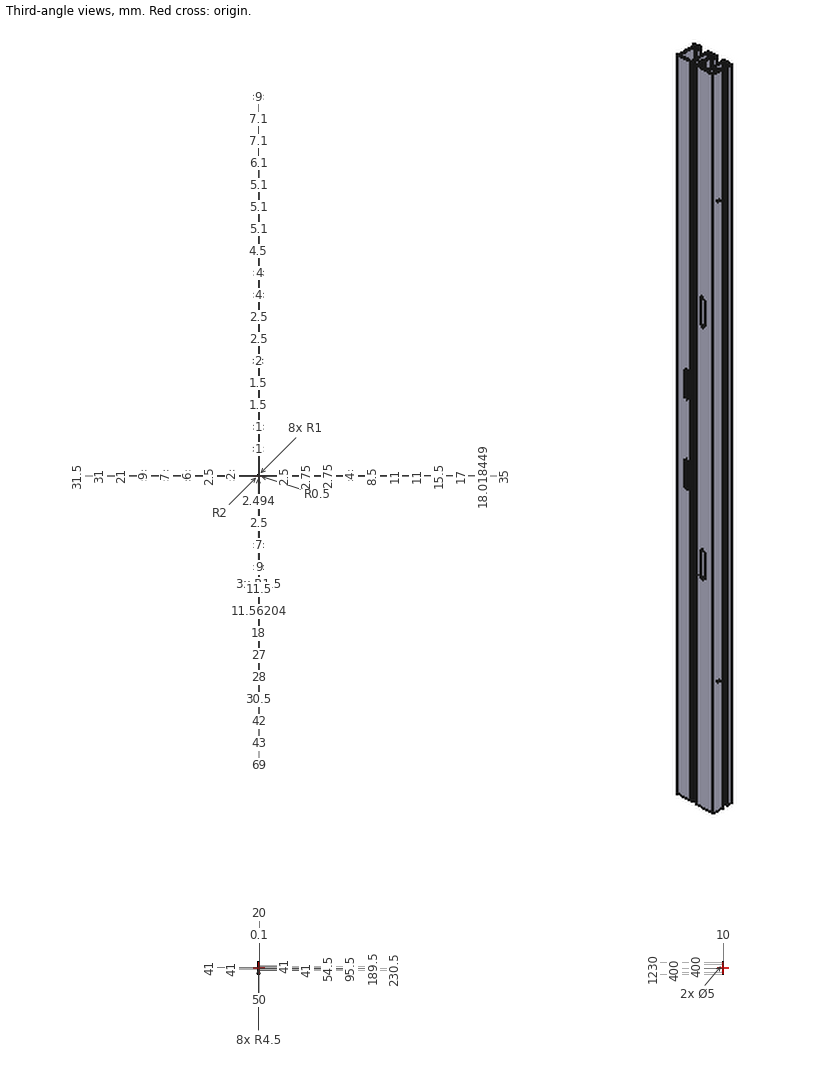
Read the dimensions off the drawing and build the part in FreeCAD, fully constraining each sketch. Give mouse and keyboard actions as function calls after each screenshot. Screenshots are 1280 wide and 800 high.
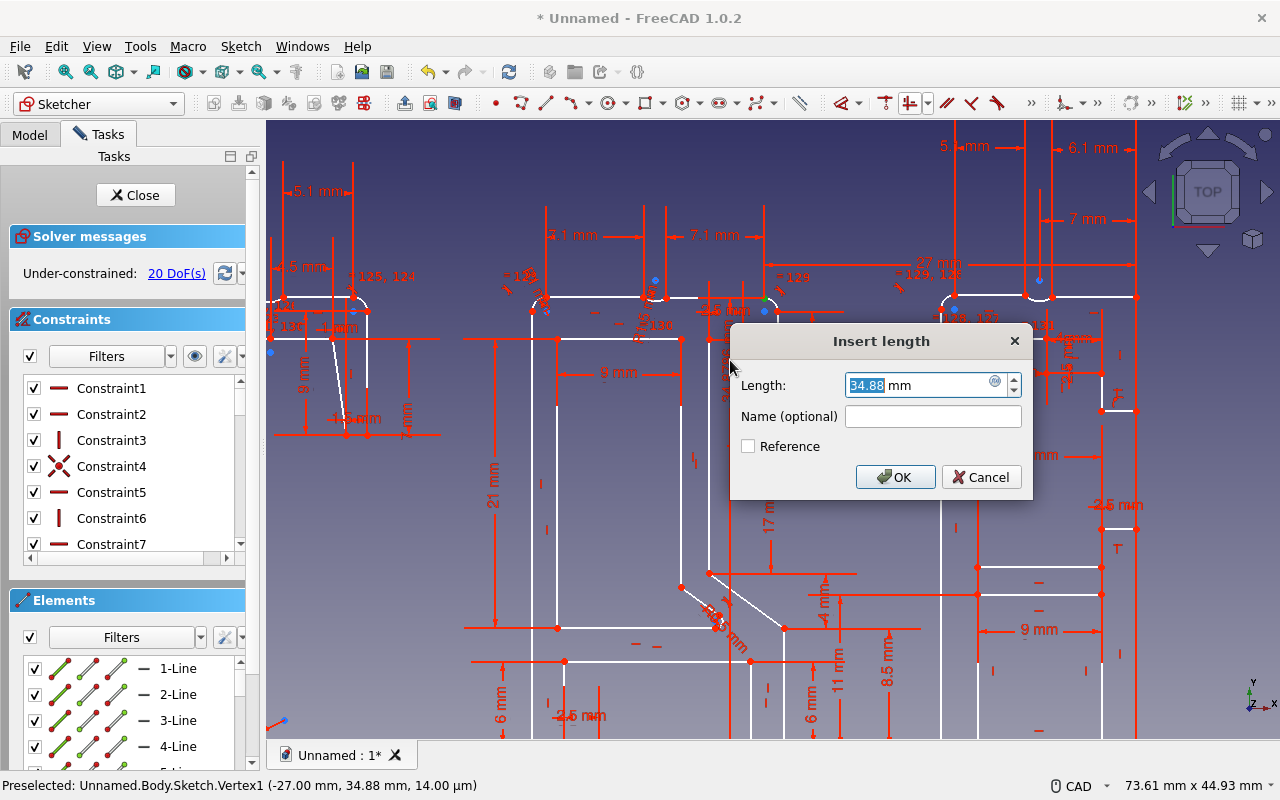
text(35)
key(Return)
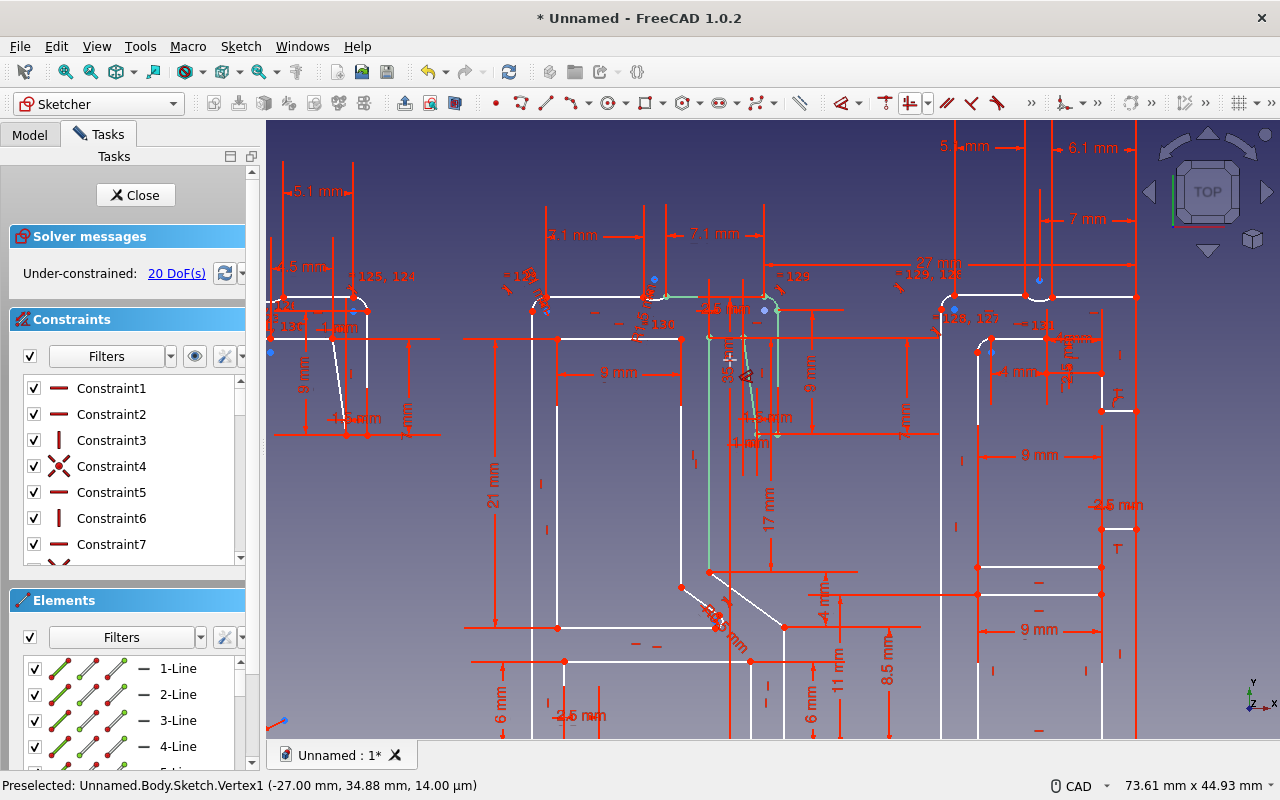
click(644, 297)
click(610, 504)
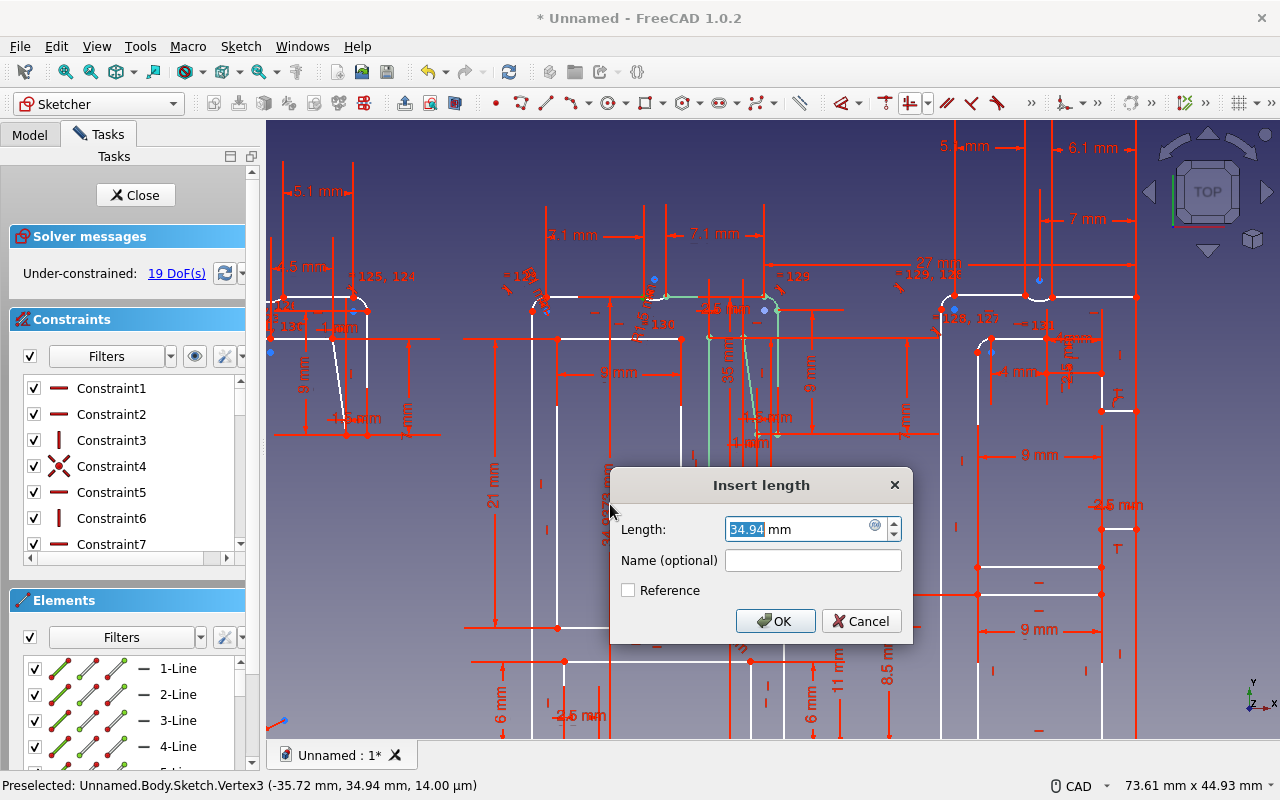
text(35)
key(Return)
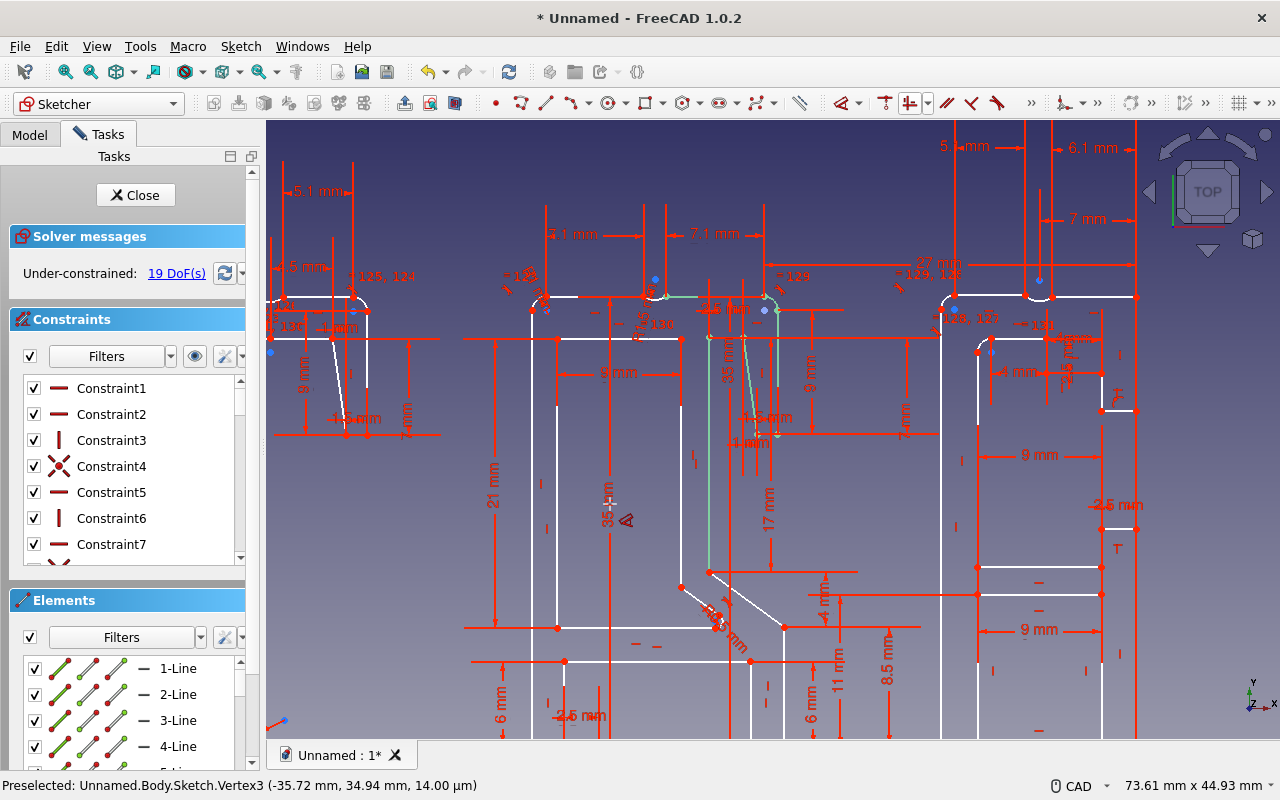
click(546, 297)
click(831, 263)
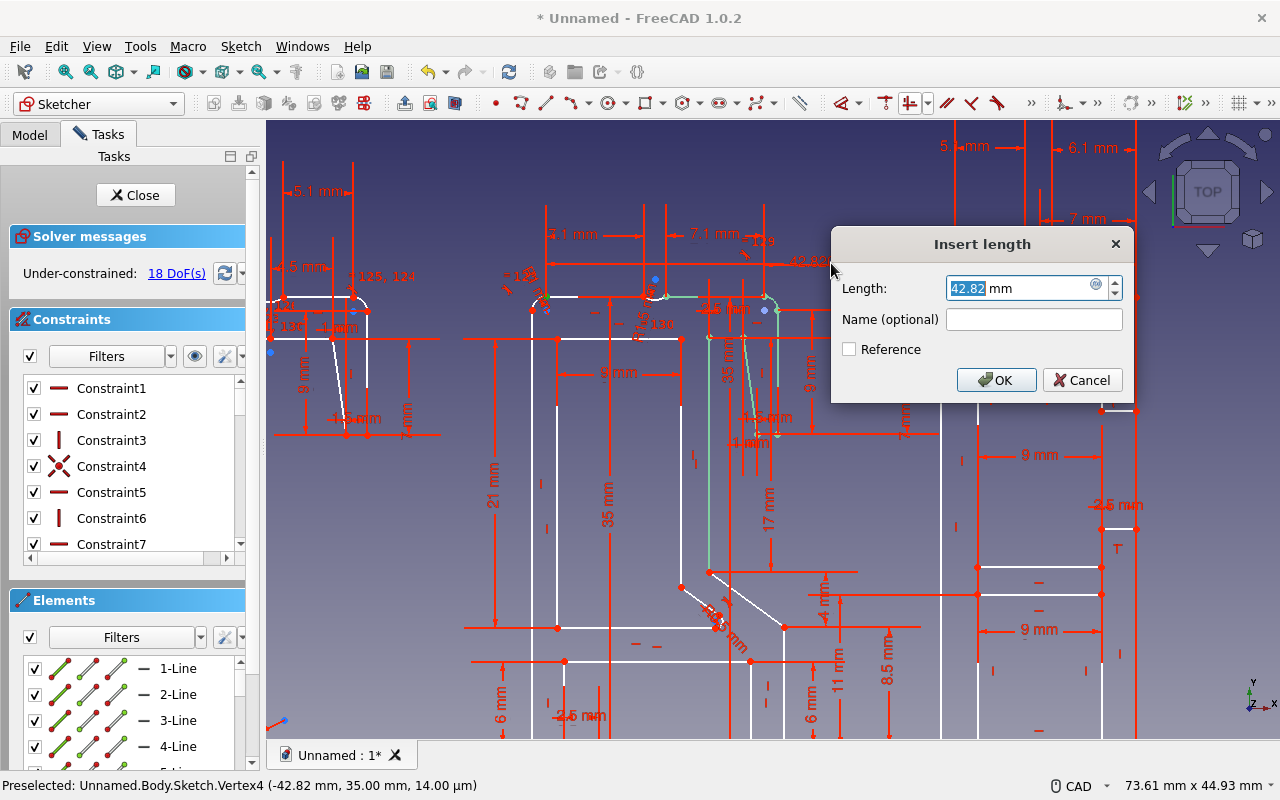
text(43)
key(Return)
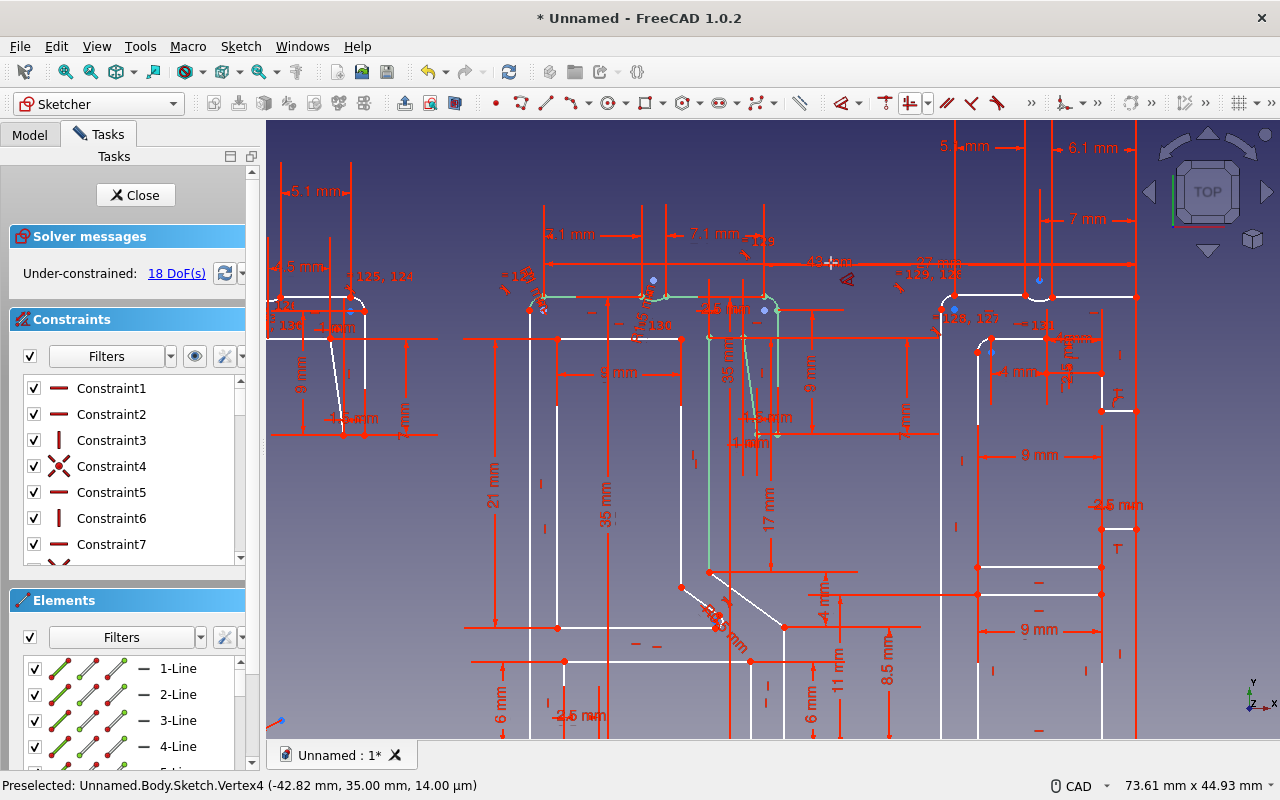
scroll(766, 298, down, 3)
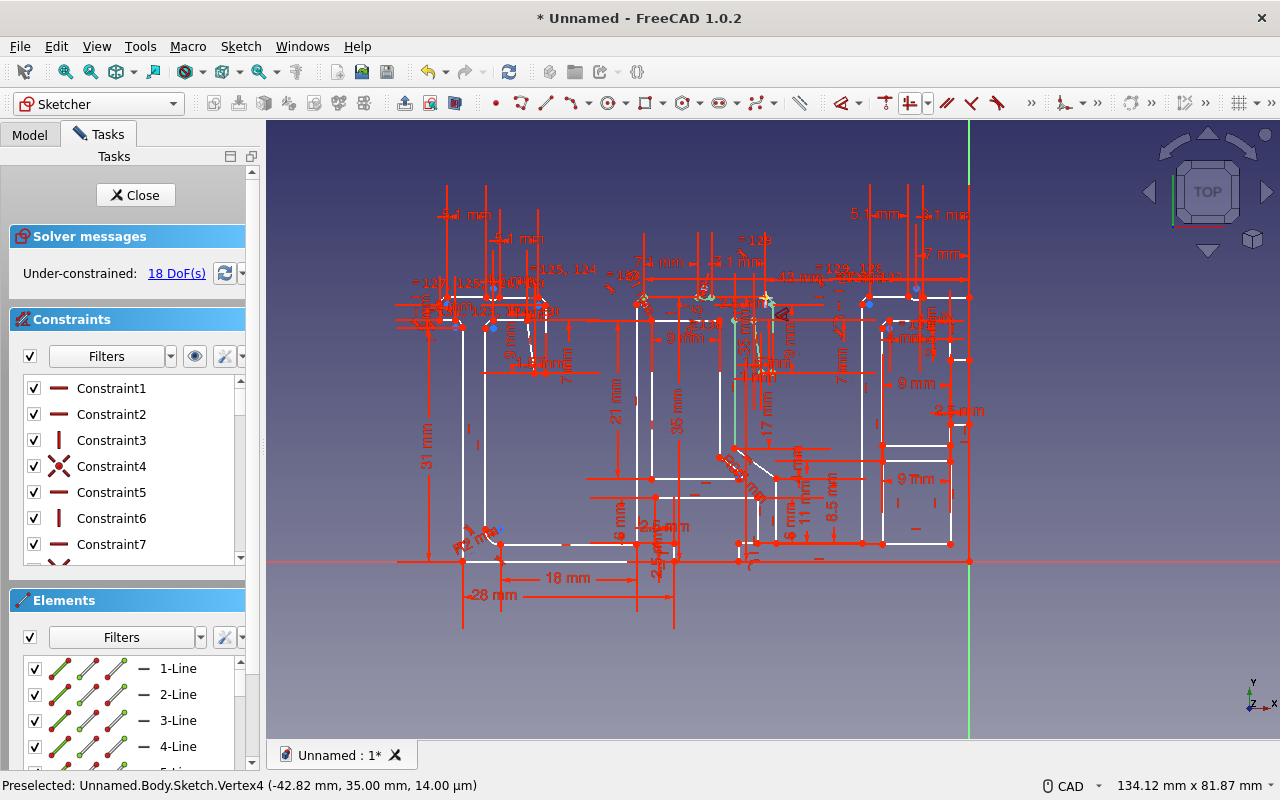
scroll(485, 328, up, 3)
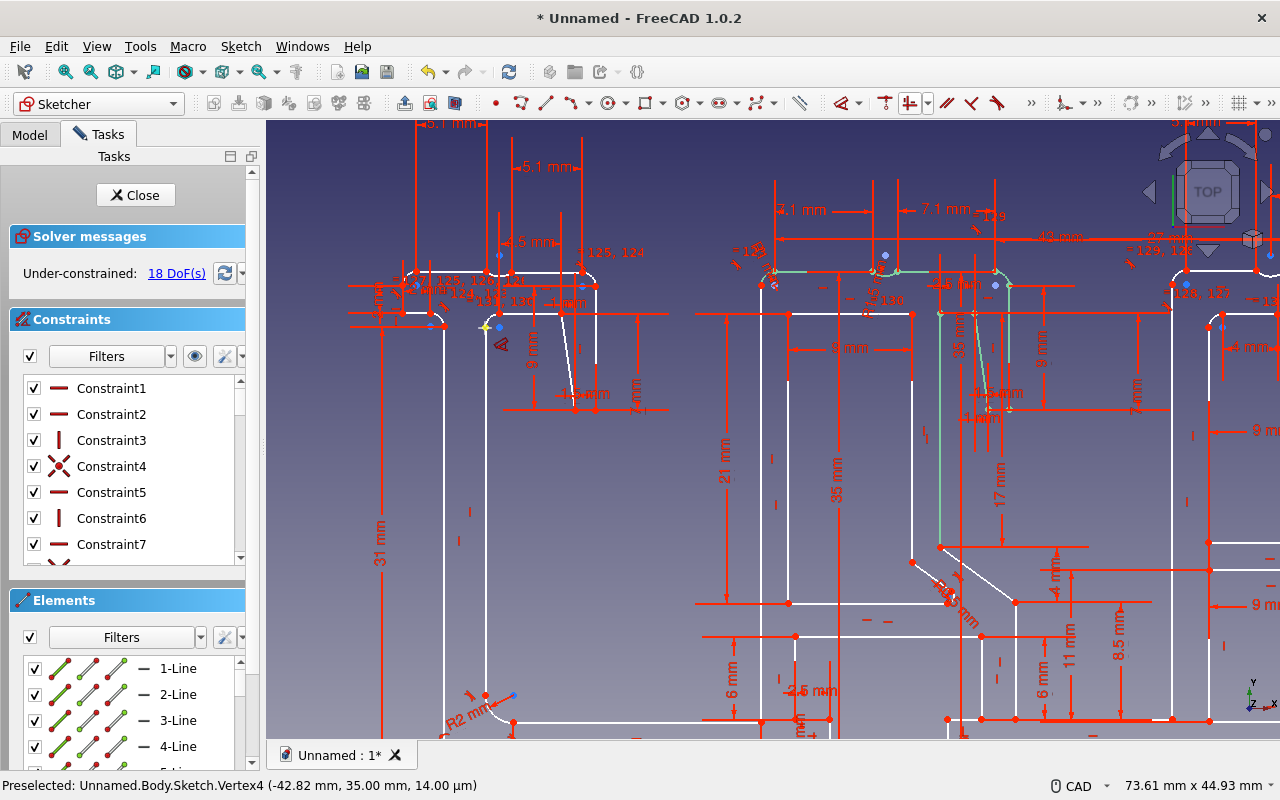
click(486, 328)
click(428, 519)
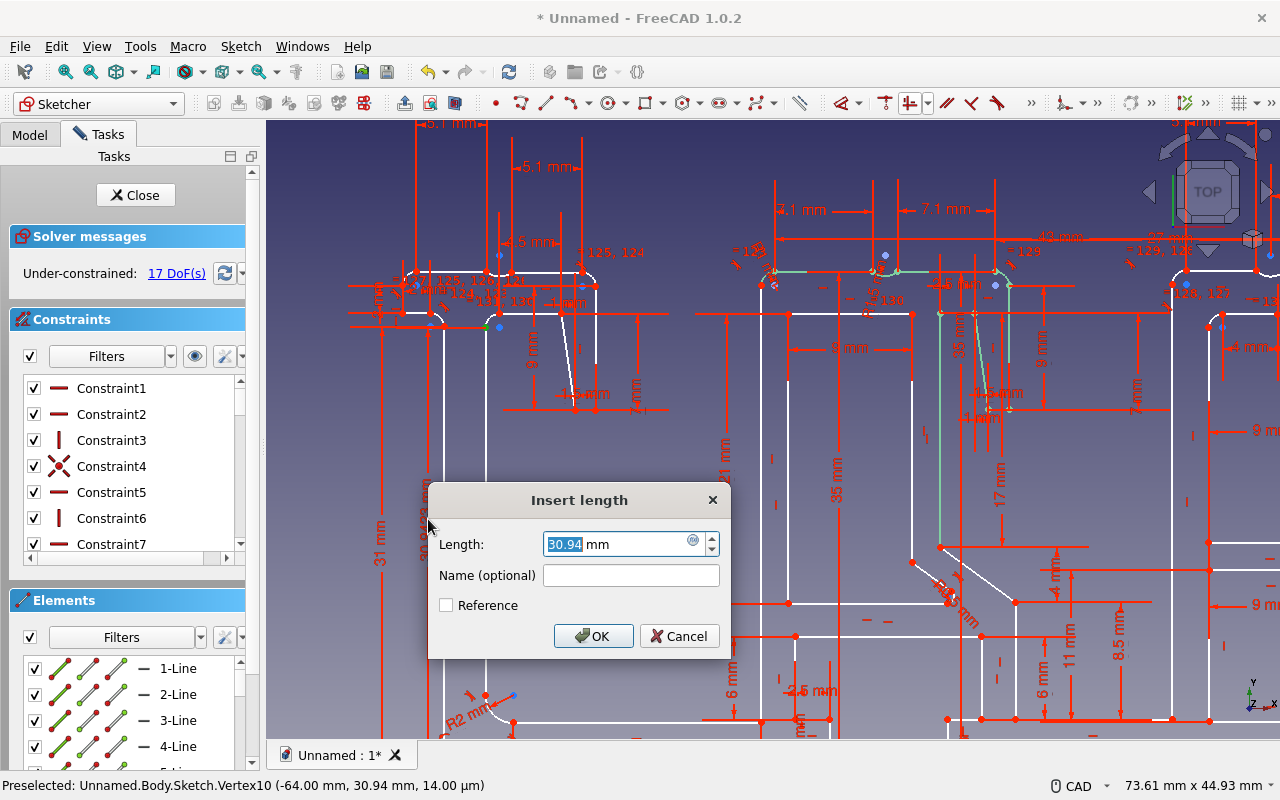
text(31)
key(Return)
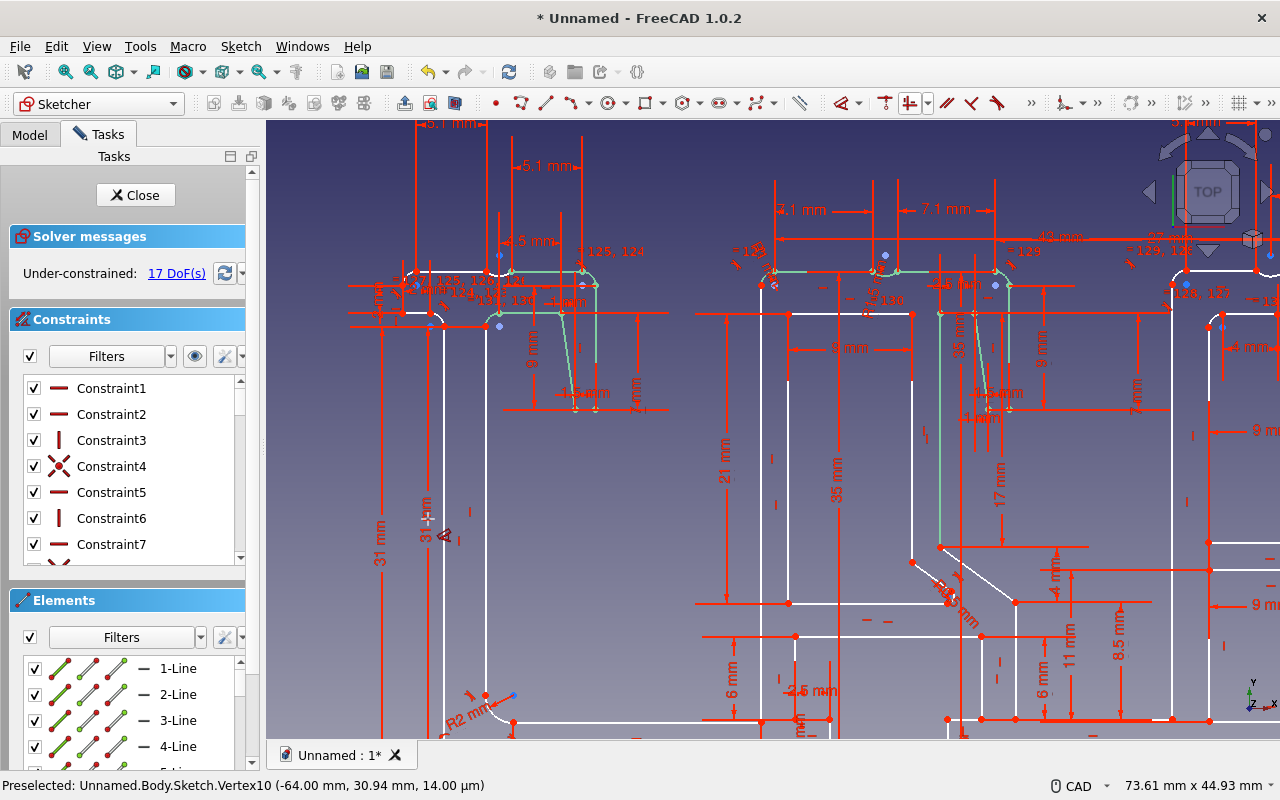
click(416, 272)
click(766, 238)